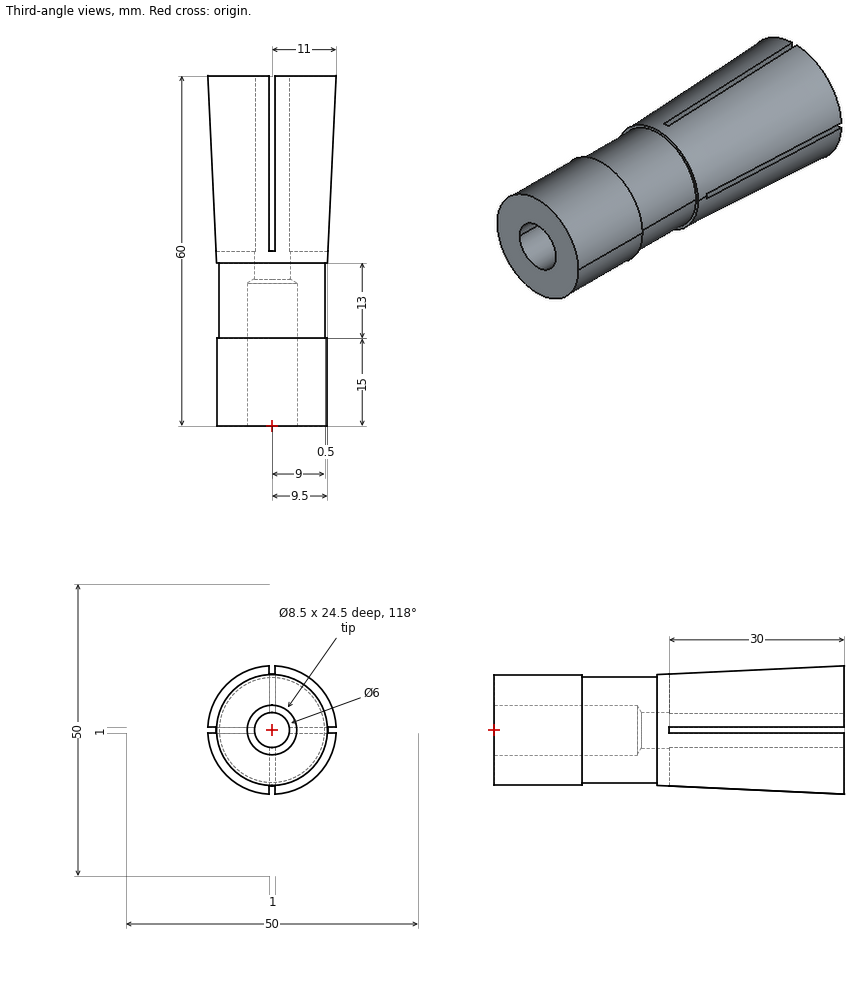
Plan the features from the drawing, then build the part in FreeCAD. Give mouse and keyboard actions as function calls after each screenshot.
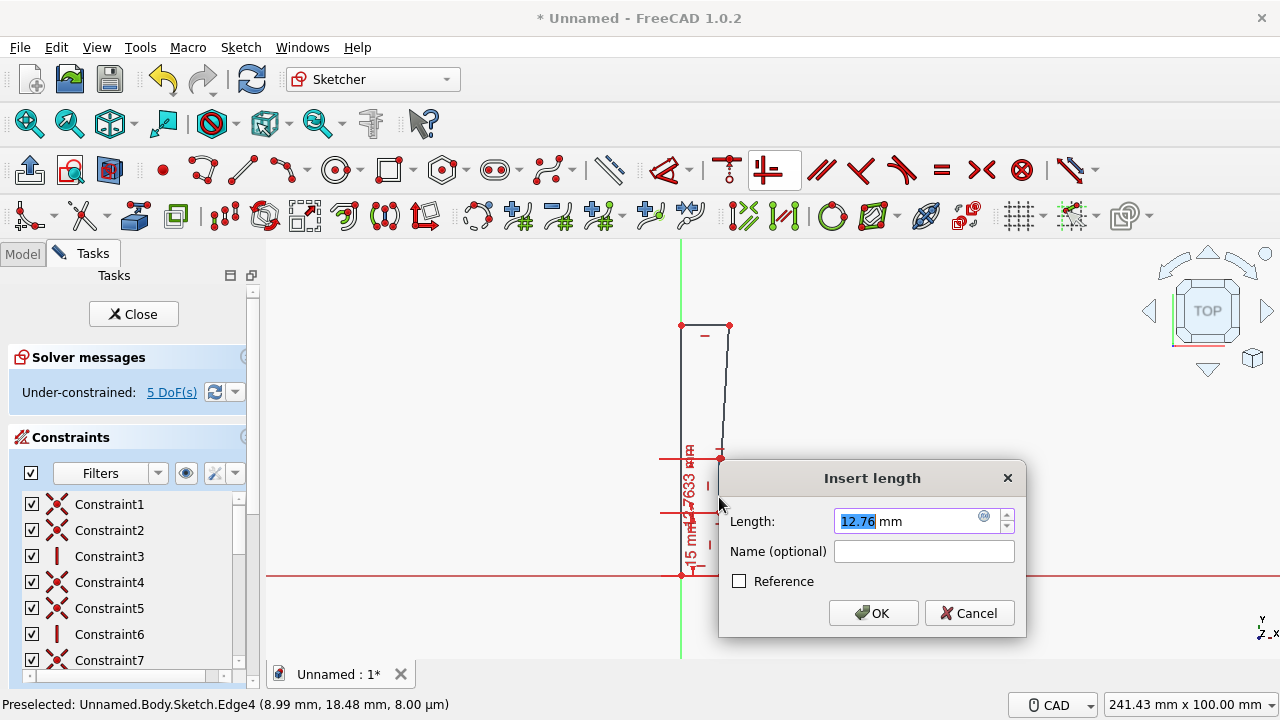
text(13)
key(Return)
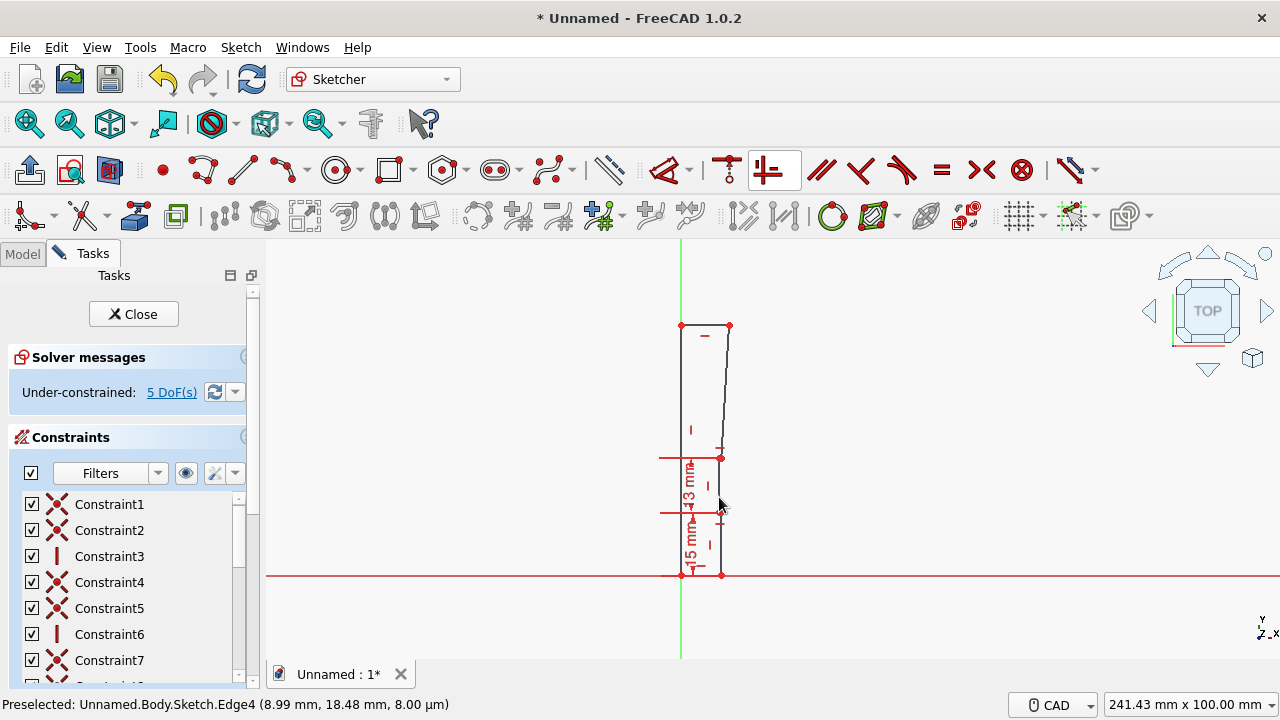
click(715, 325)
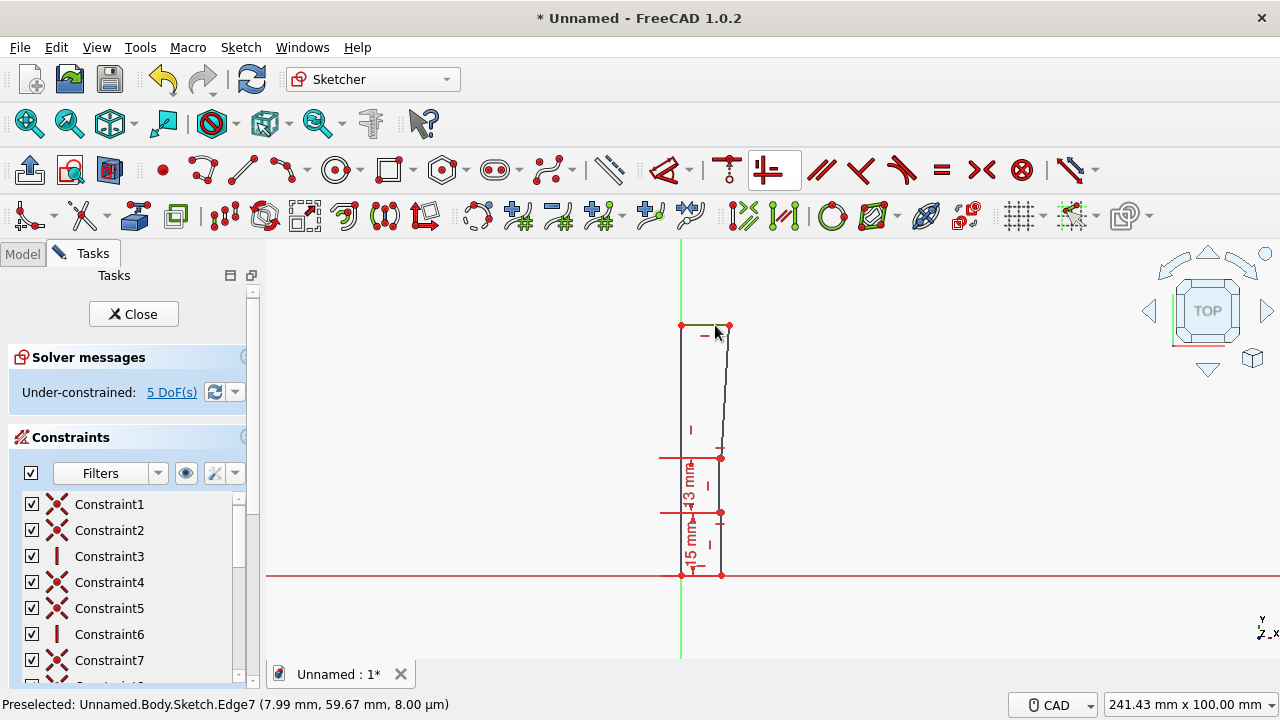
key(l)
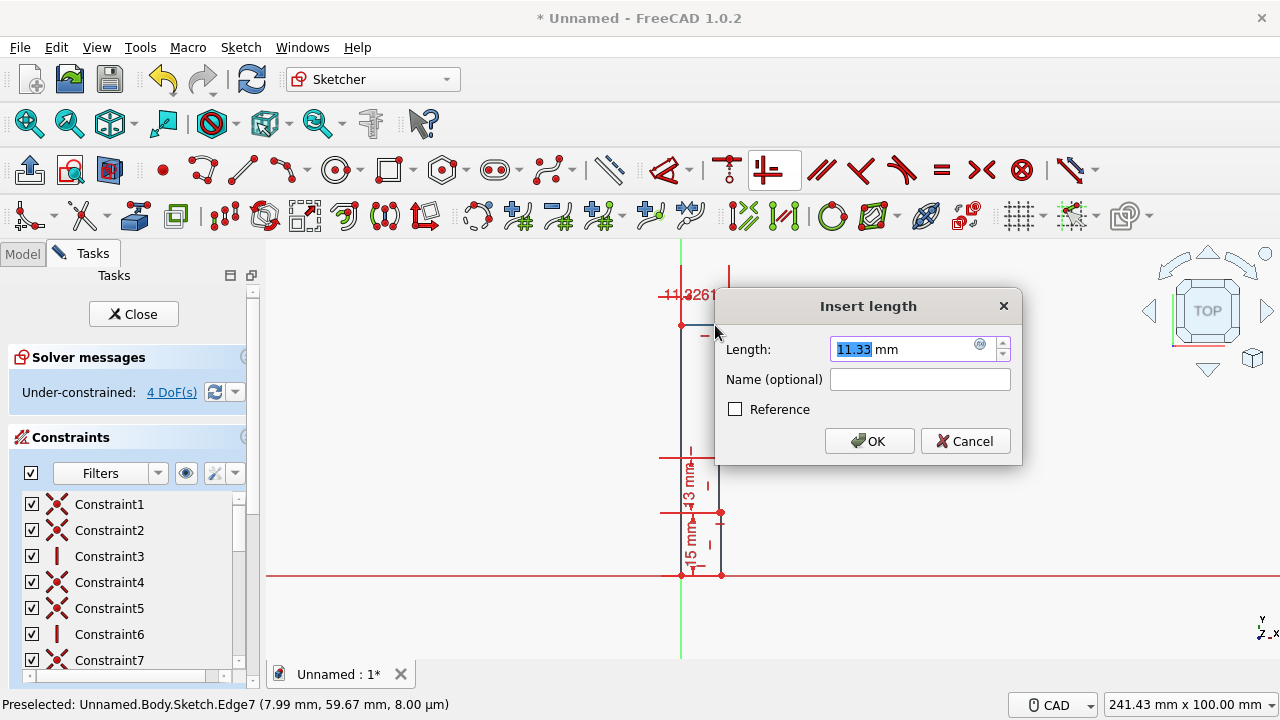
text(11)
key(Return)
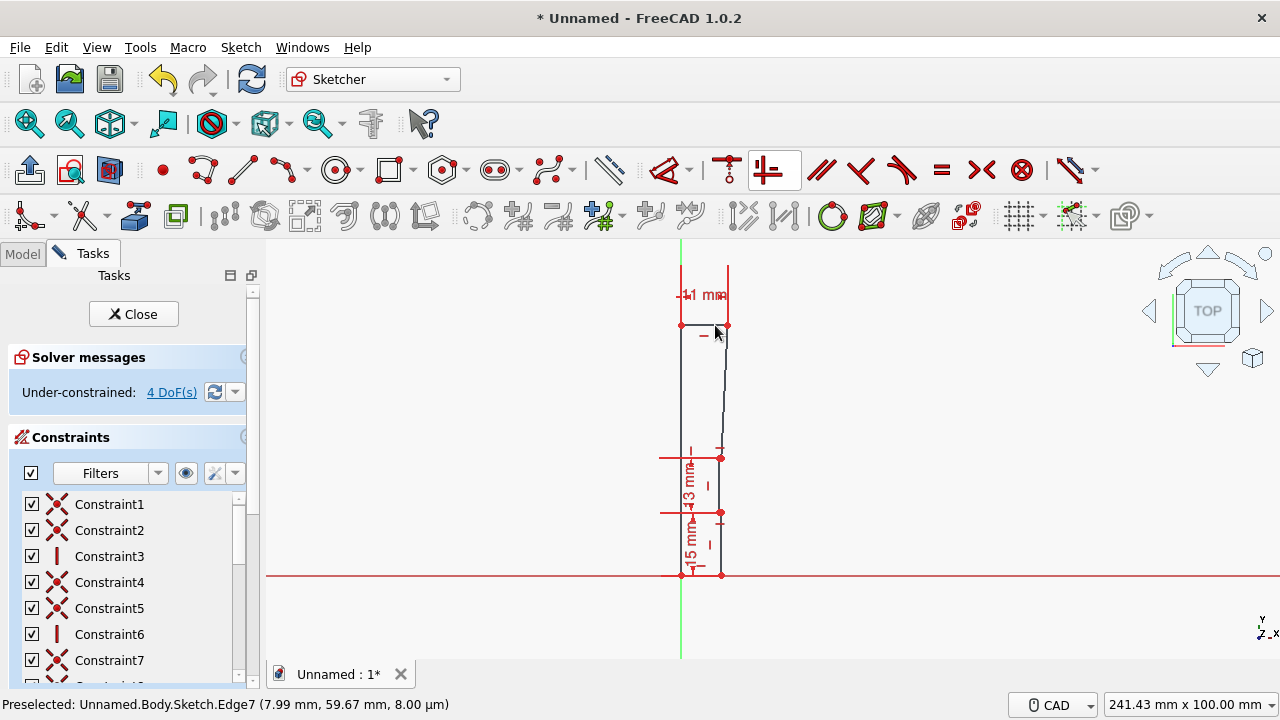
click(681, 400)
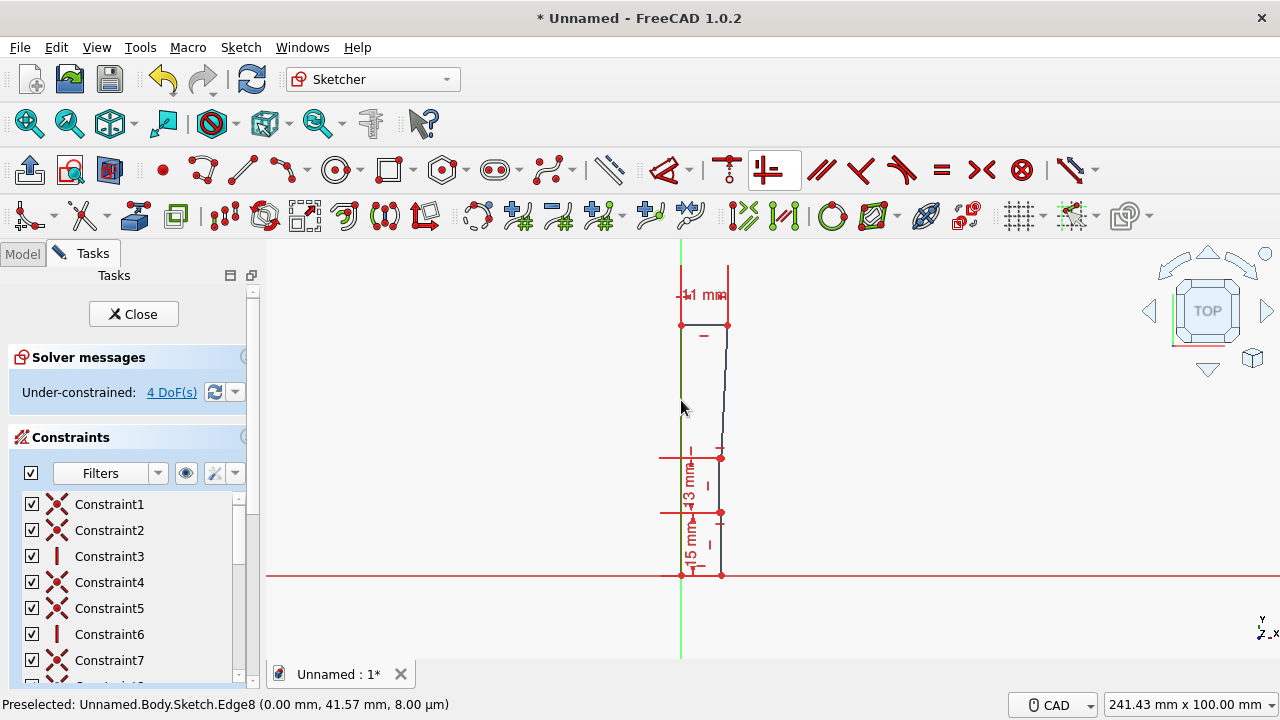
key(i)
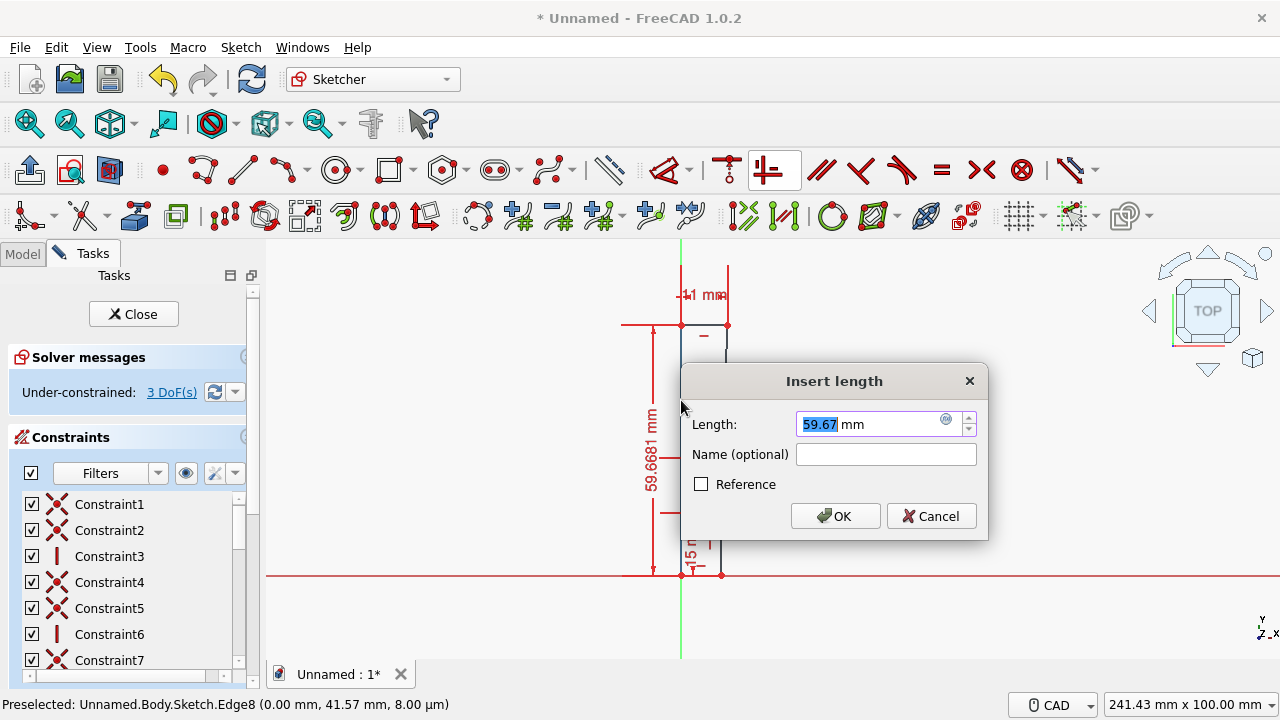
text(60)
key(Return)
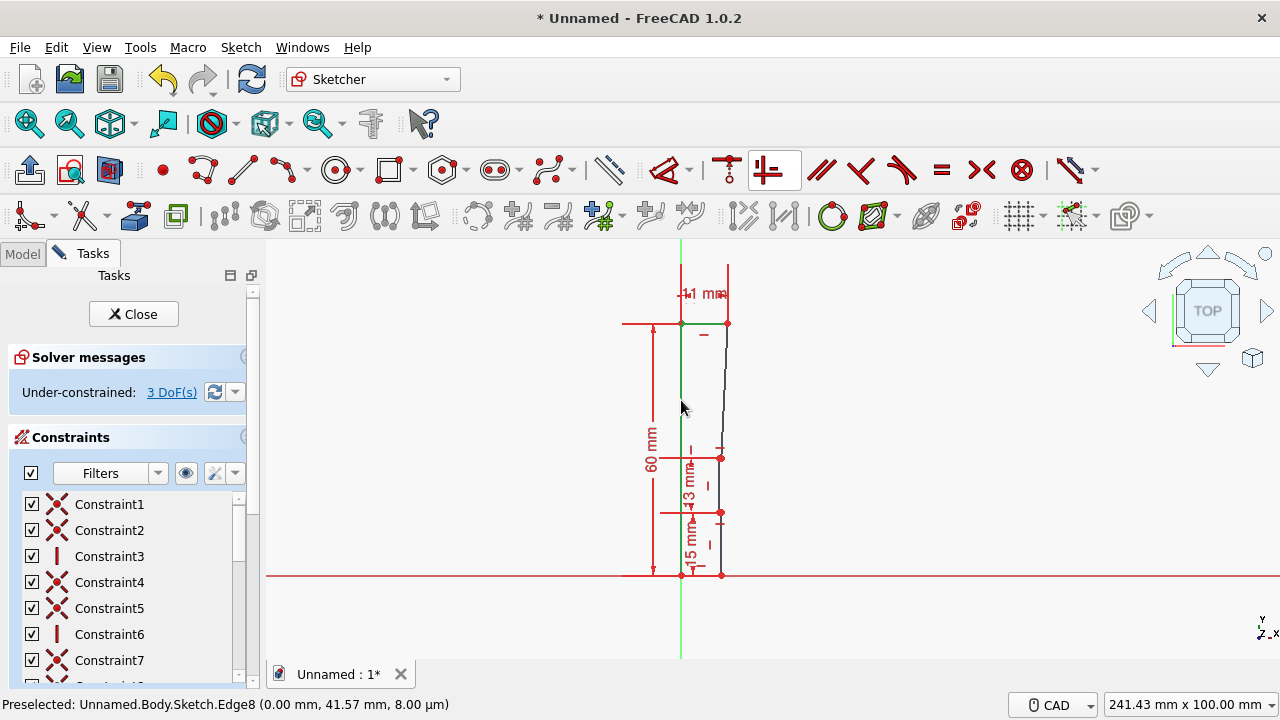
scroll(719, 513, up, 10)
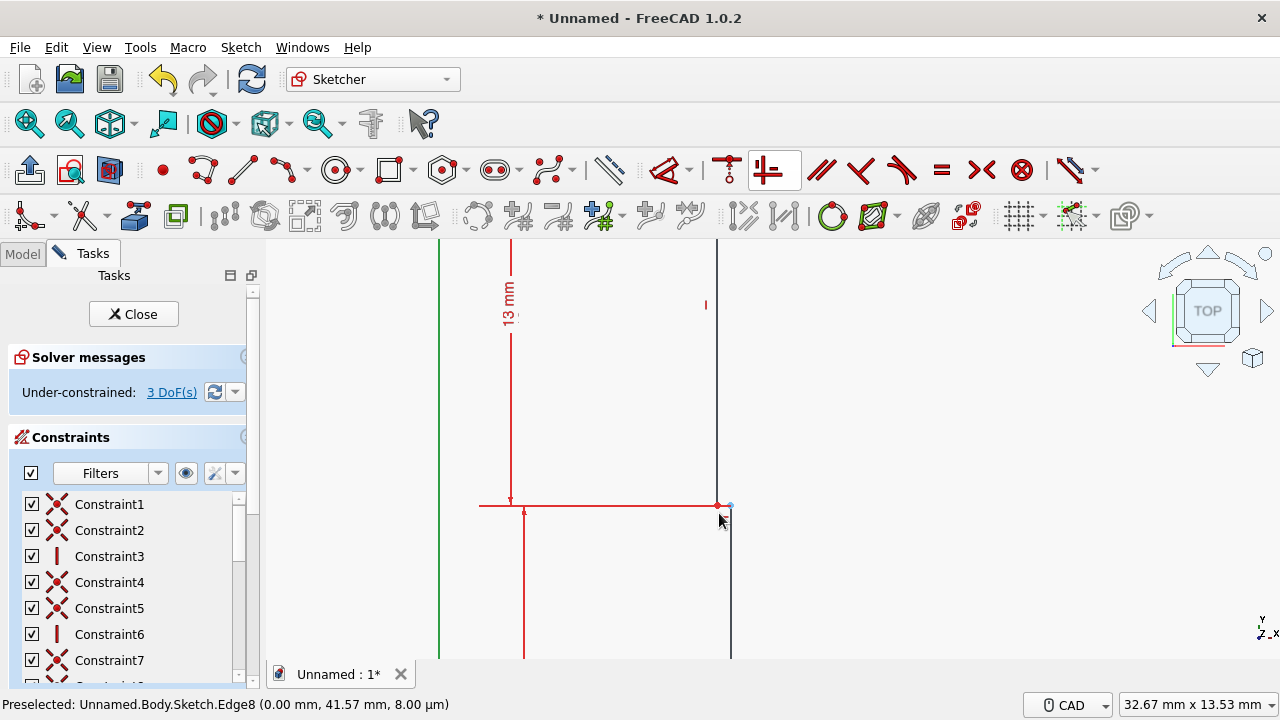
click(717, 506)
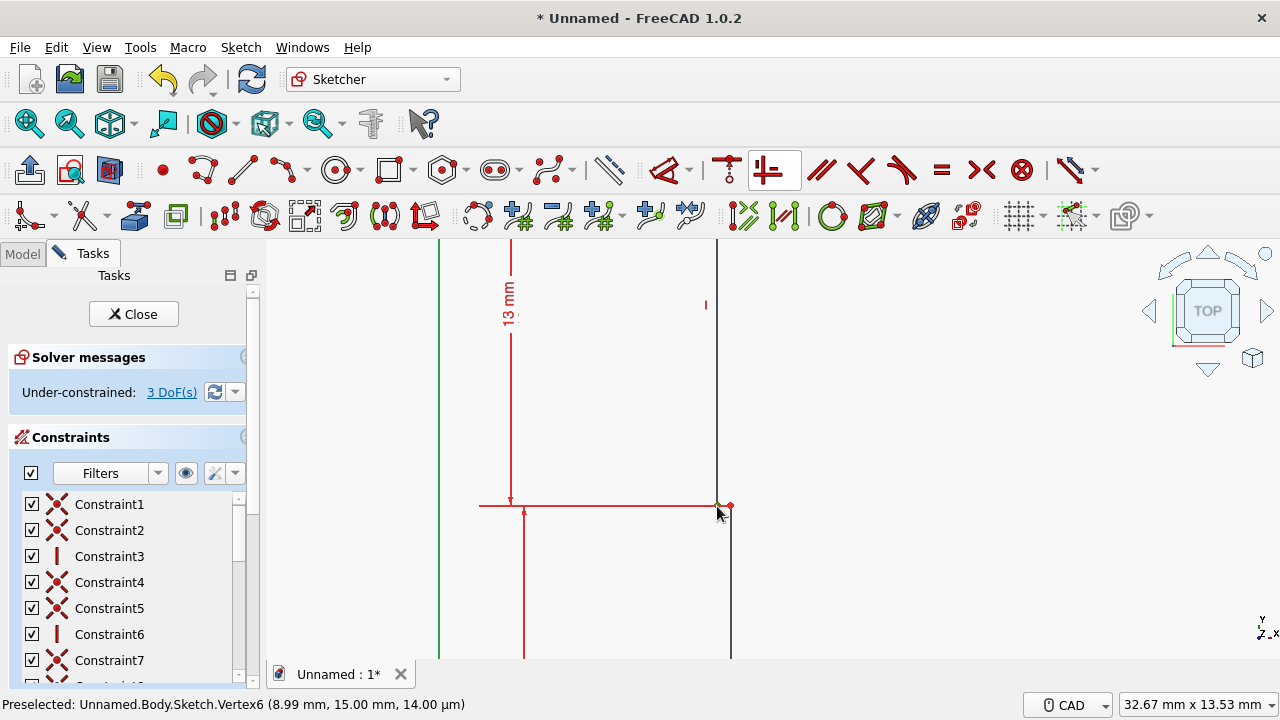
click(692, 170)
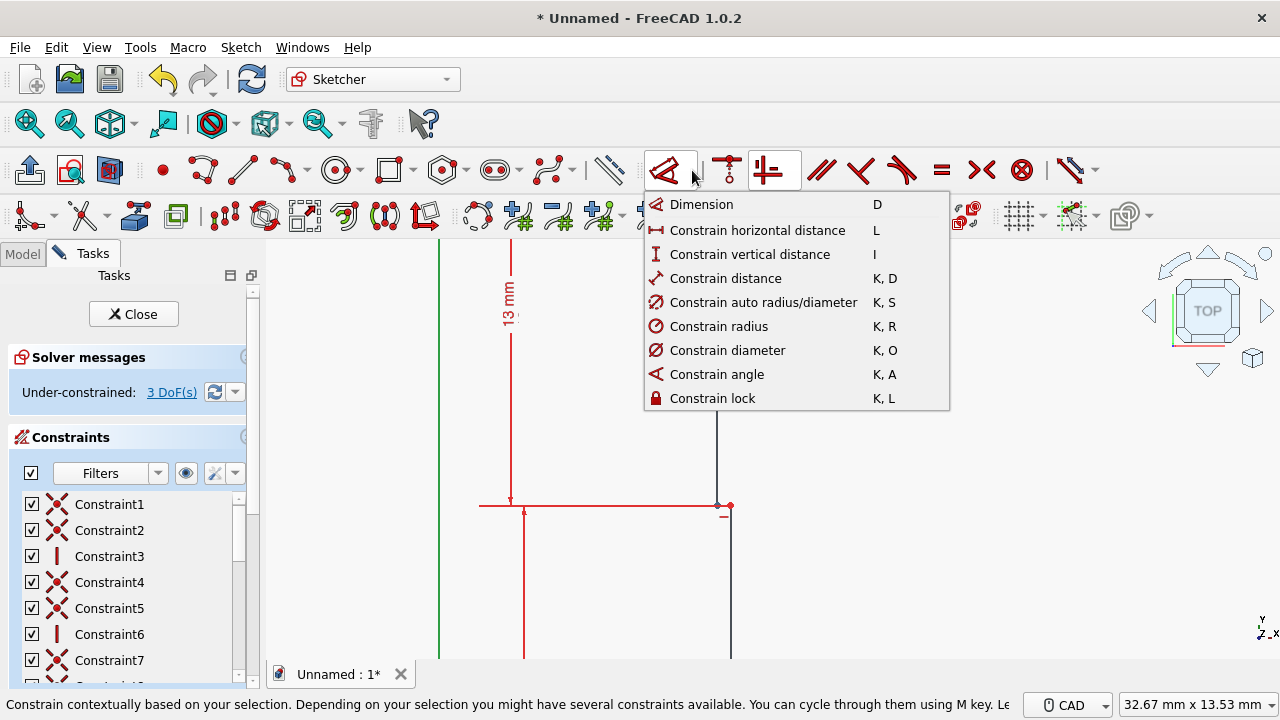
click(797, 230)